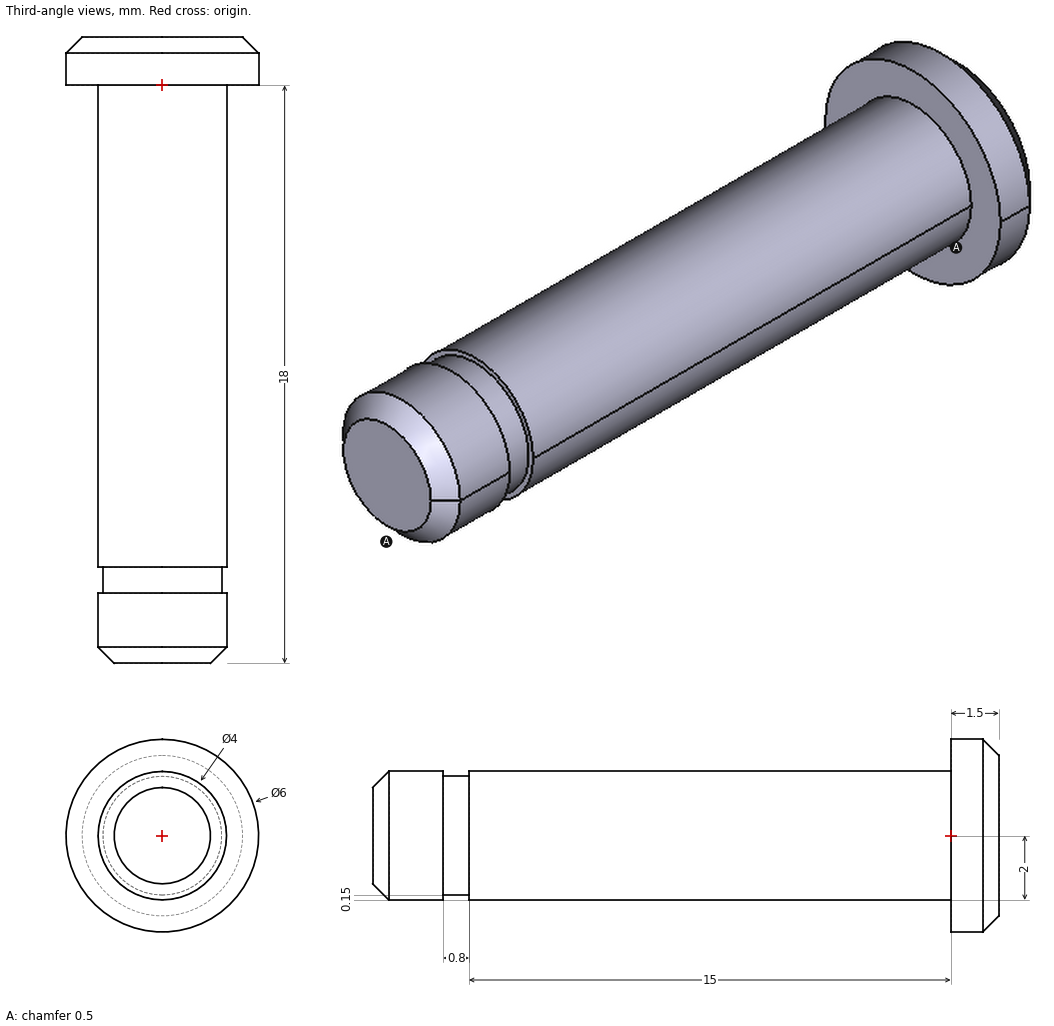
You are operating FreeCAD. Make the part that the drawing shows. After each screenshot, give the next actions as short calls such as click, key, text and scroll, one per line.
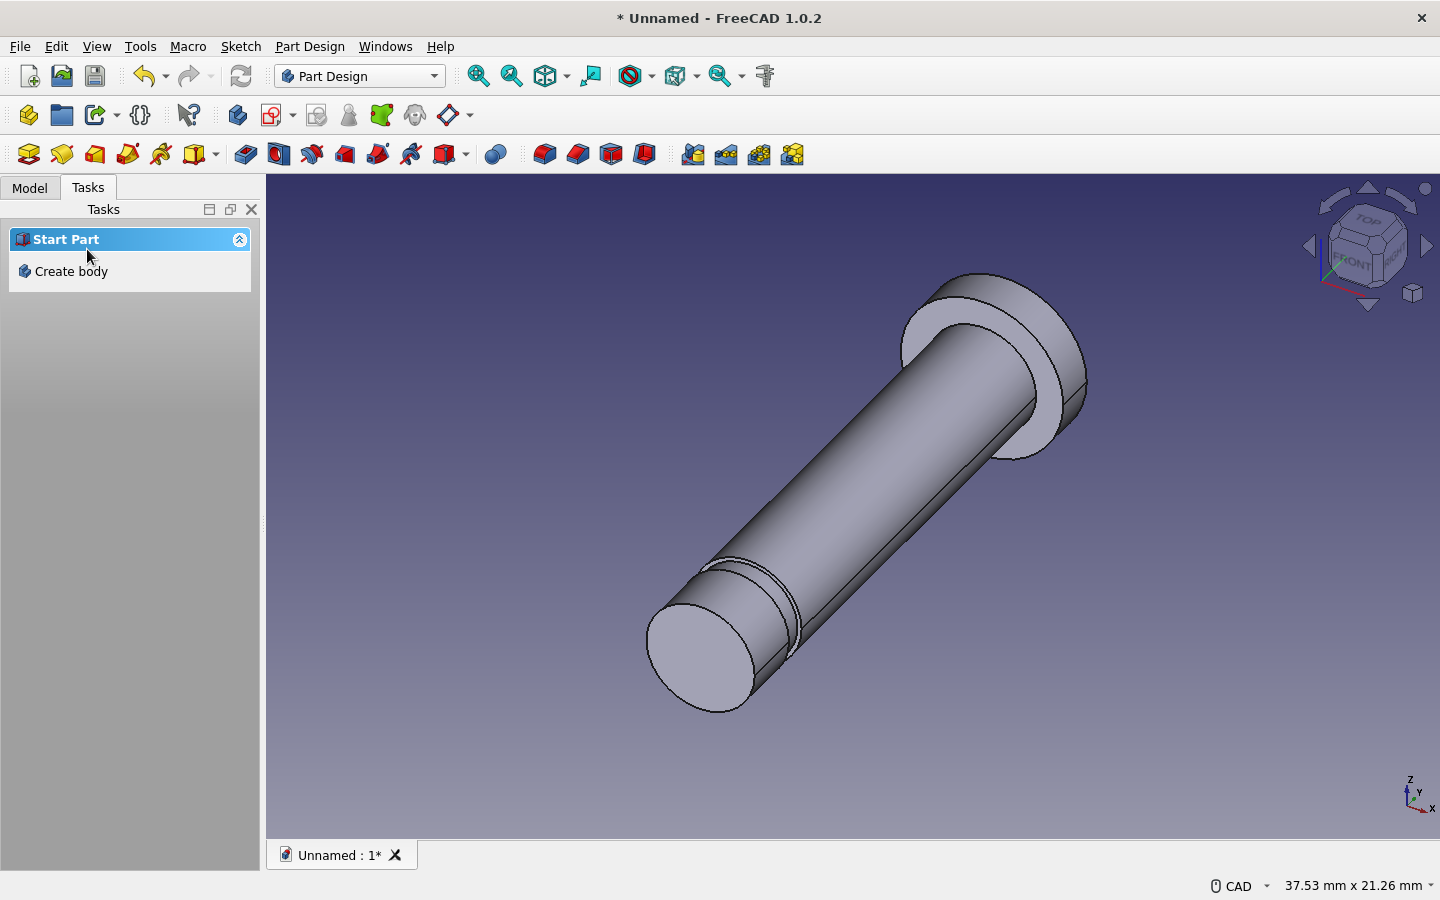
click(657, 612)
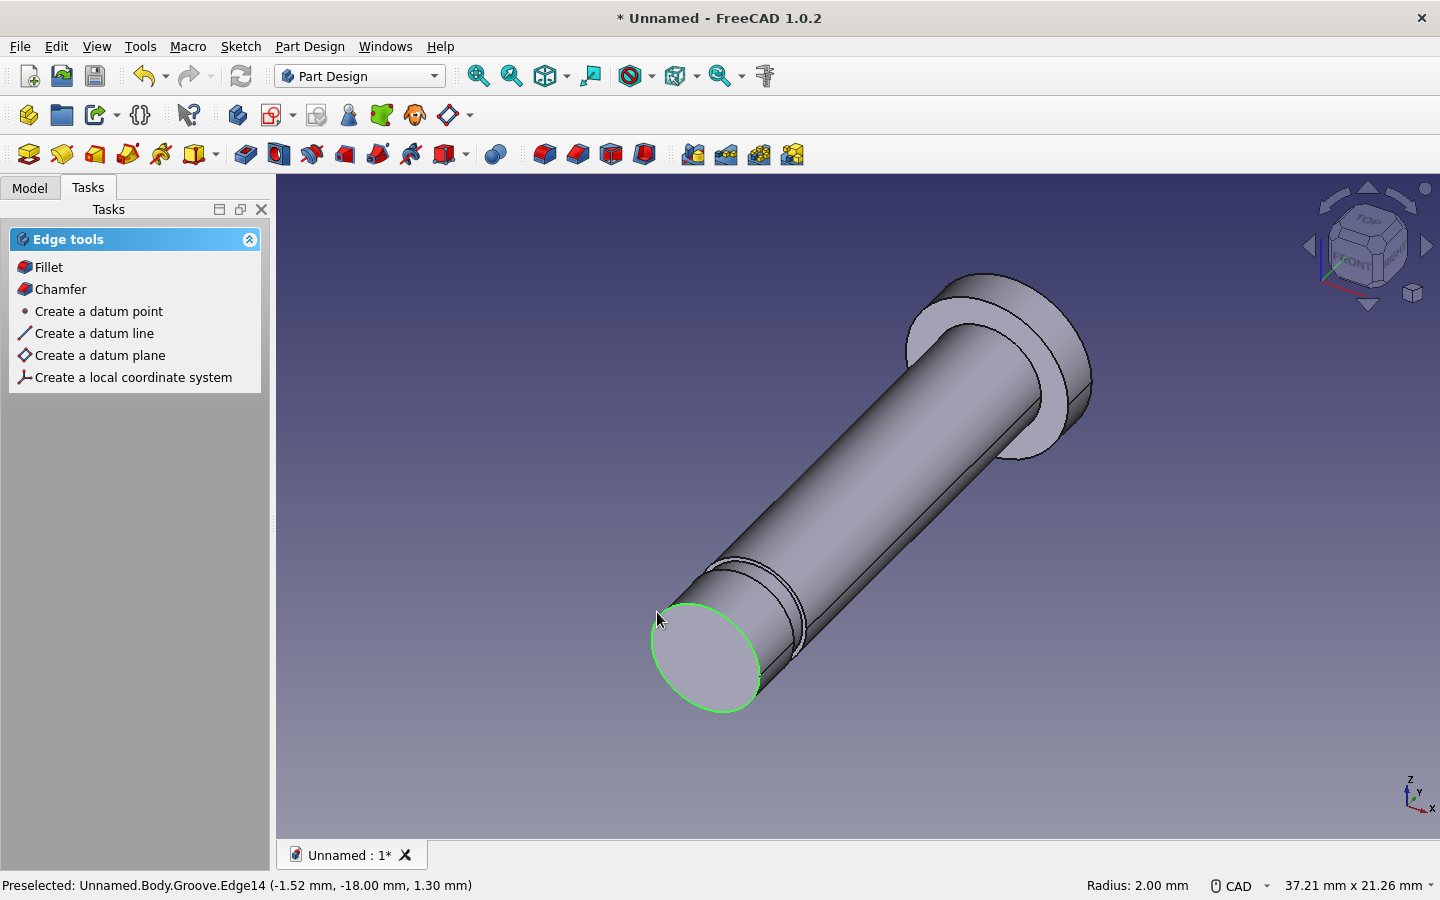
key(0)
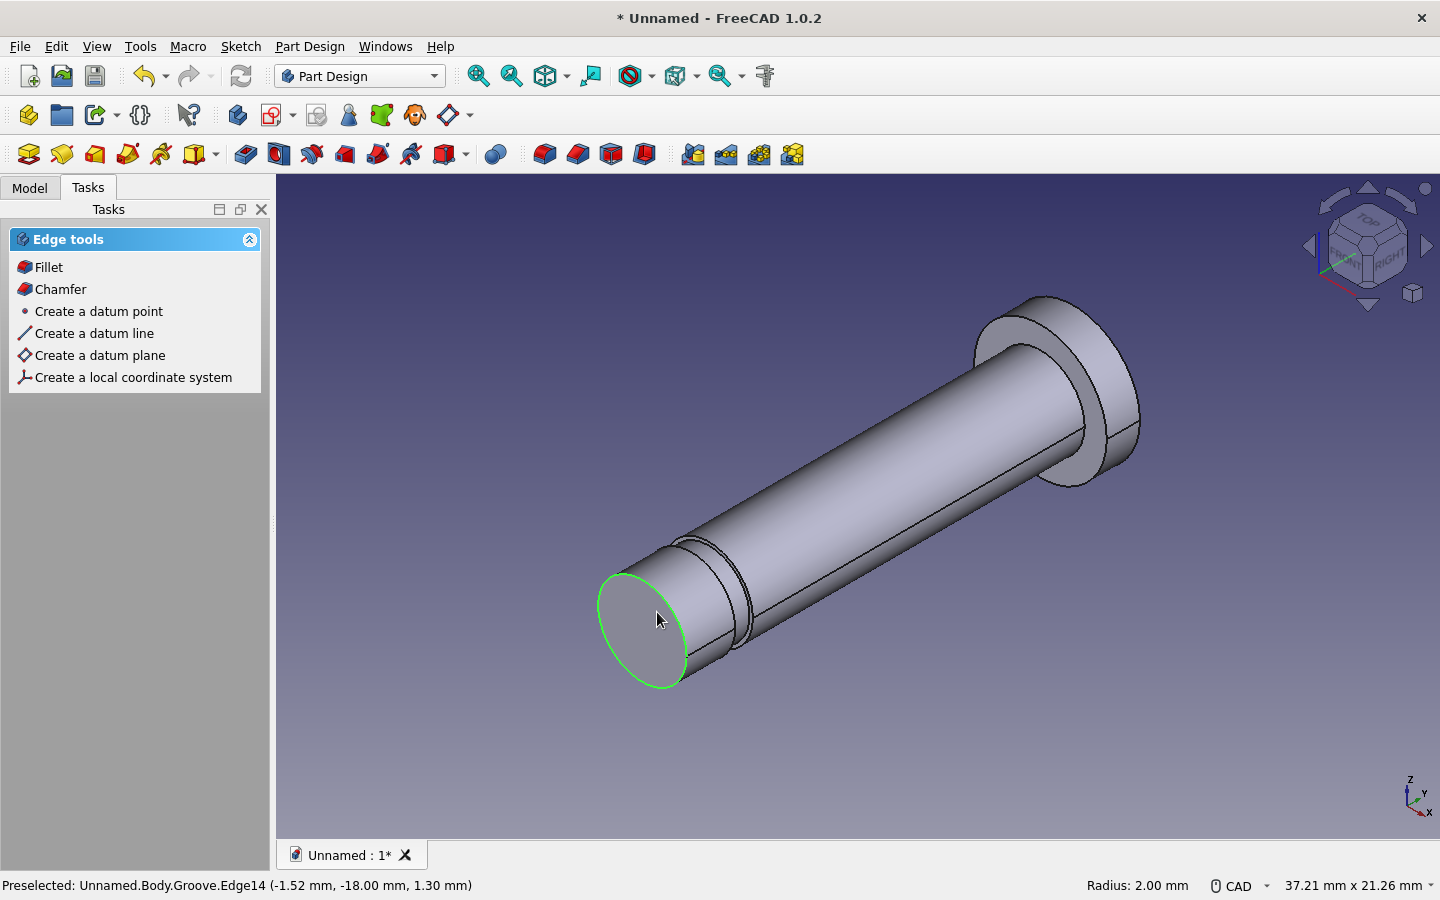
key(2)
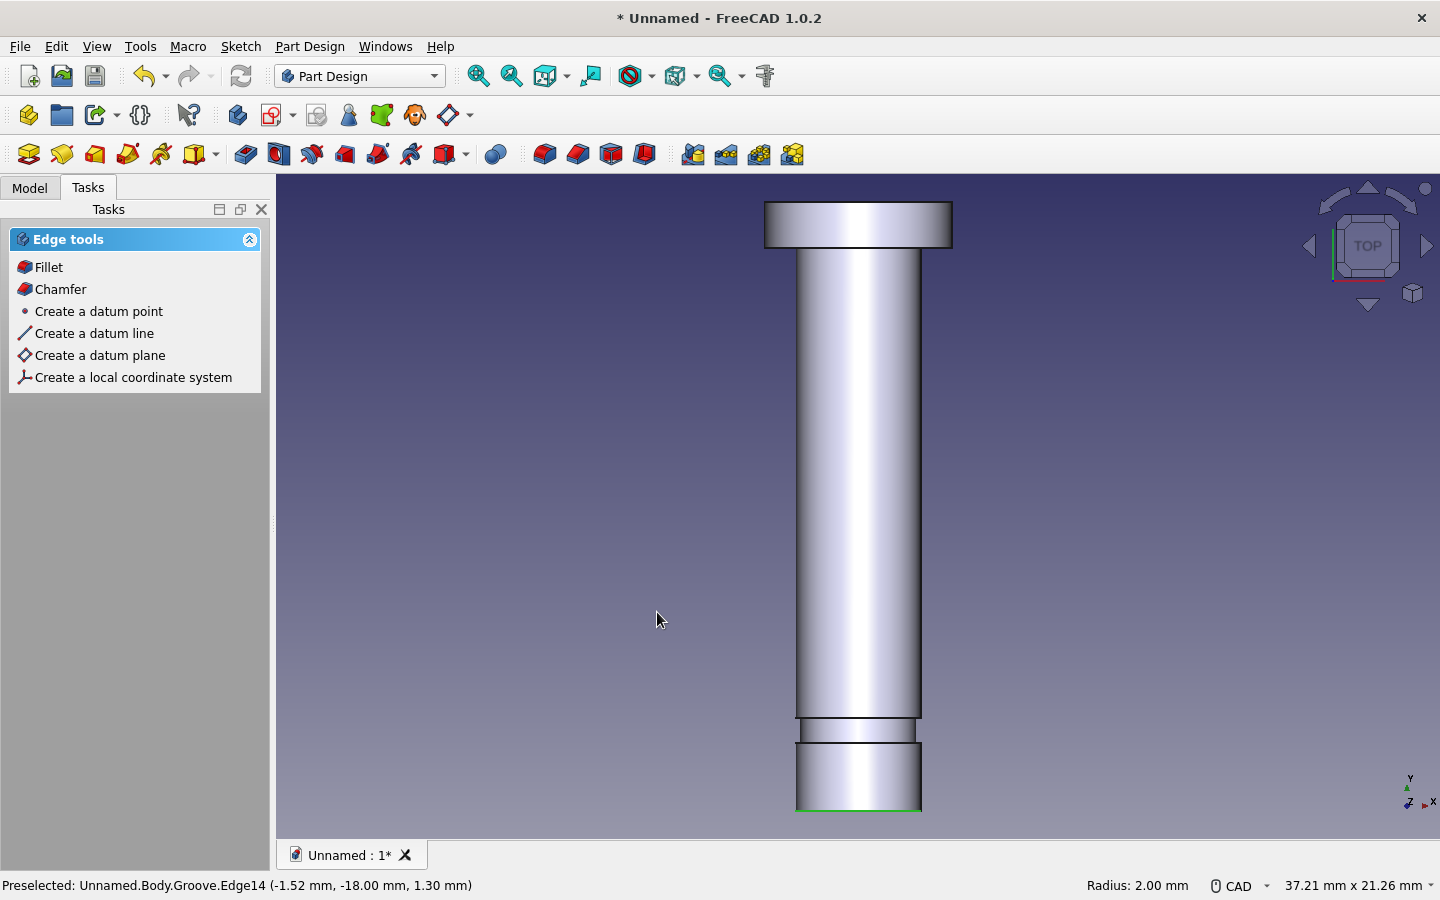
key(1)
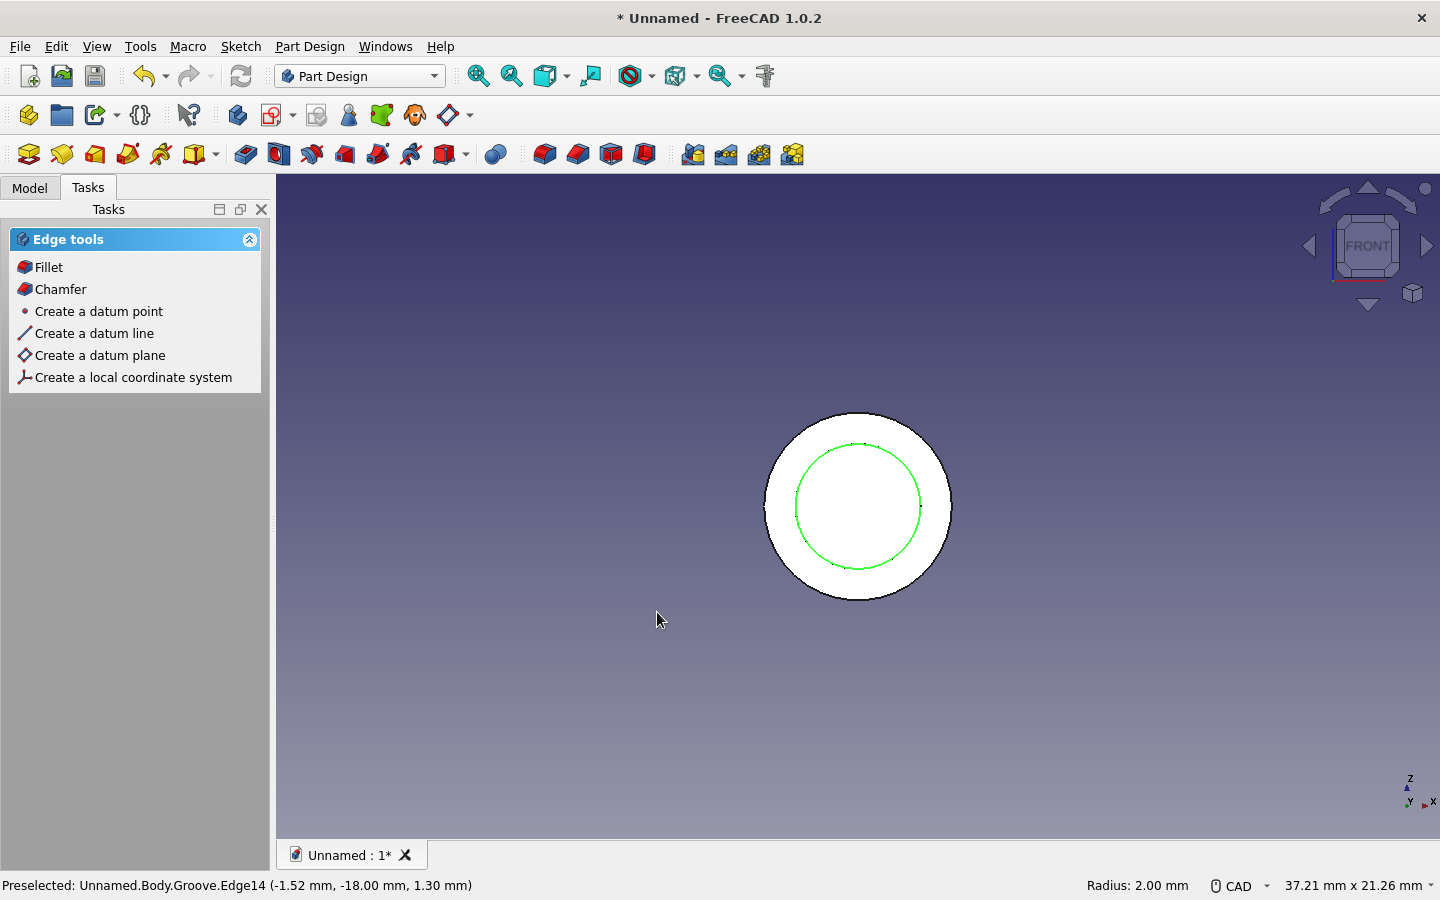
click(479, 76)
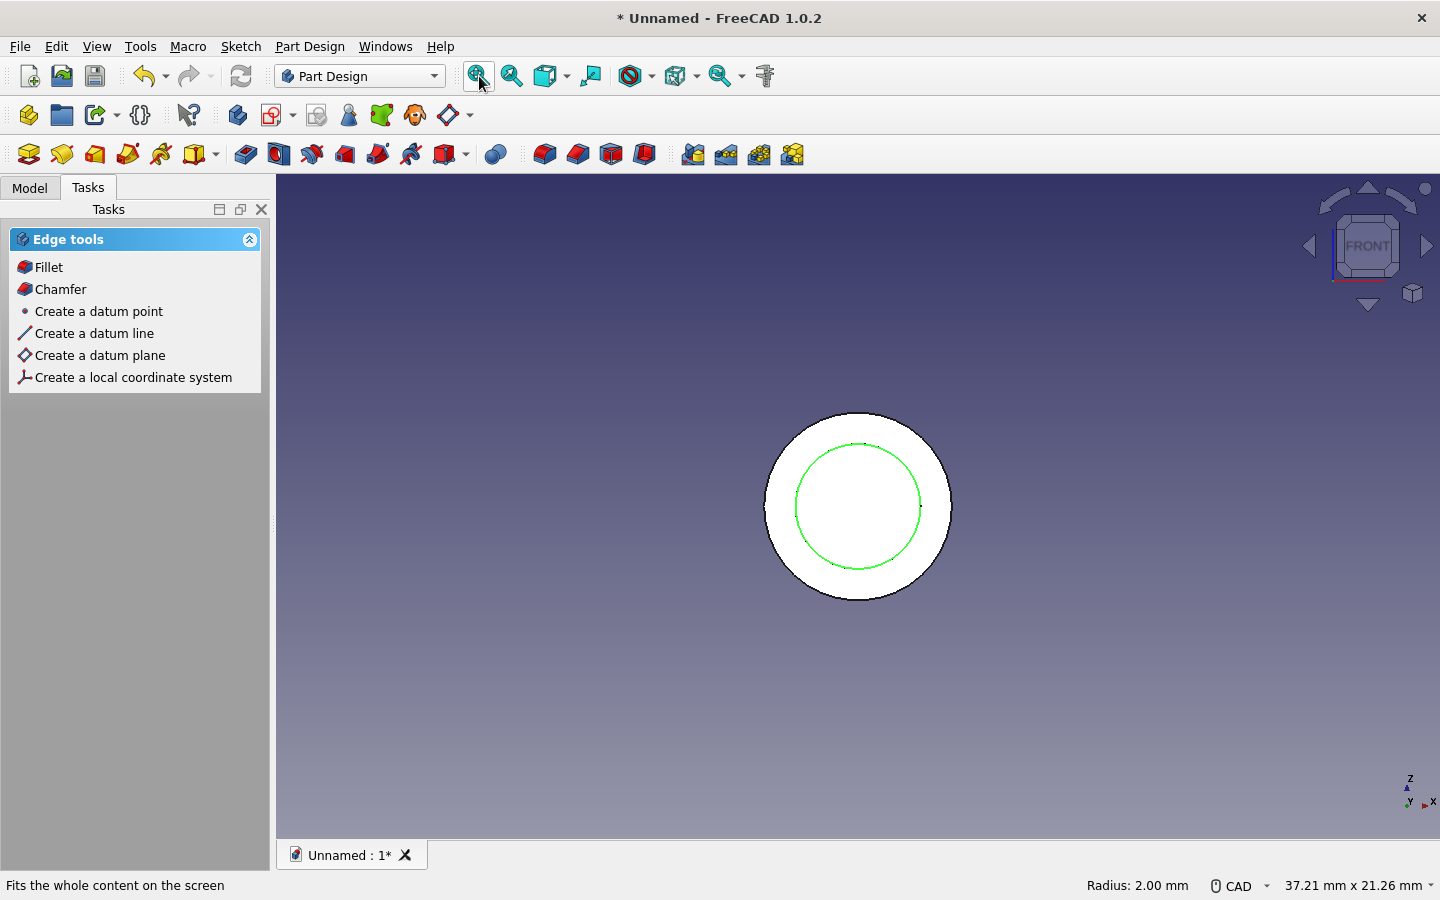
key(3)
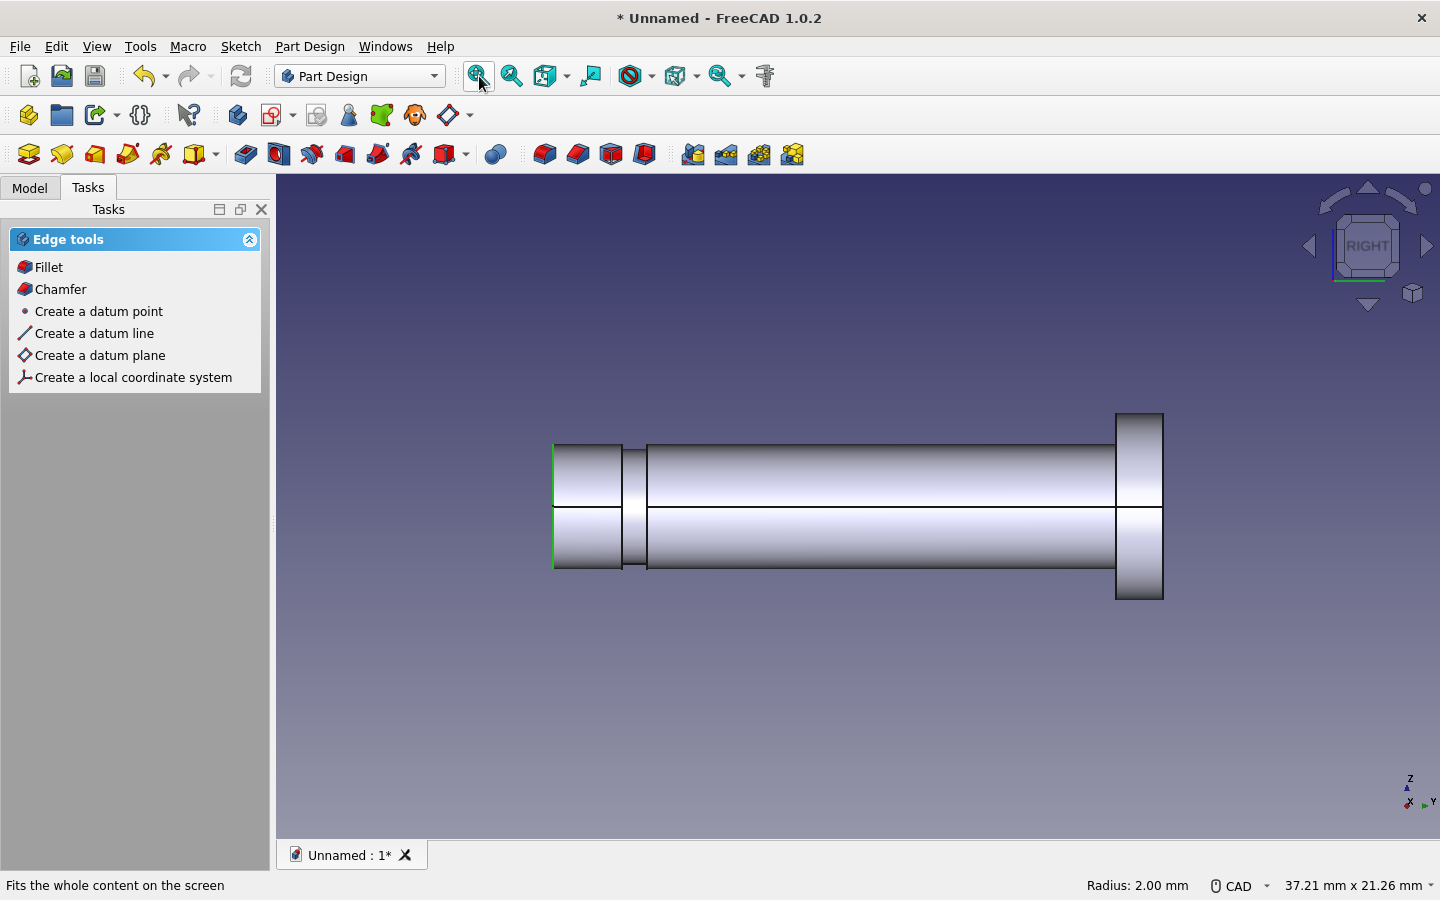
click(1163, 450, ctrl)